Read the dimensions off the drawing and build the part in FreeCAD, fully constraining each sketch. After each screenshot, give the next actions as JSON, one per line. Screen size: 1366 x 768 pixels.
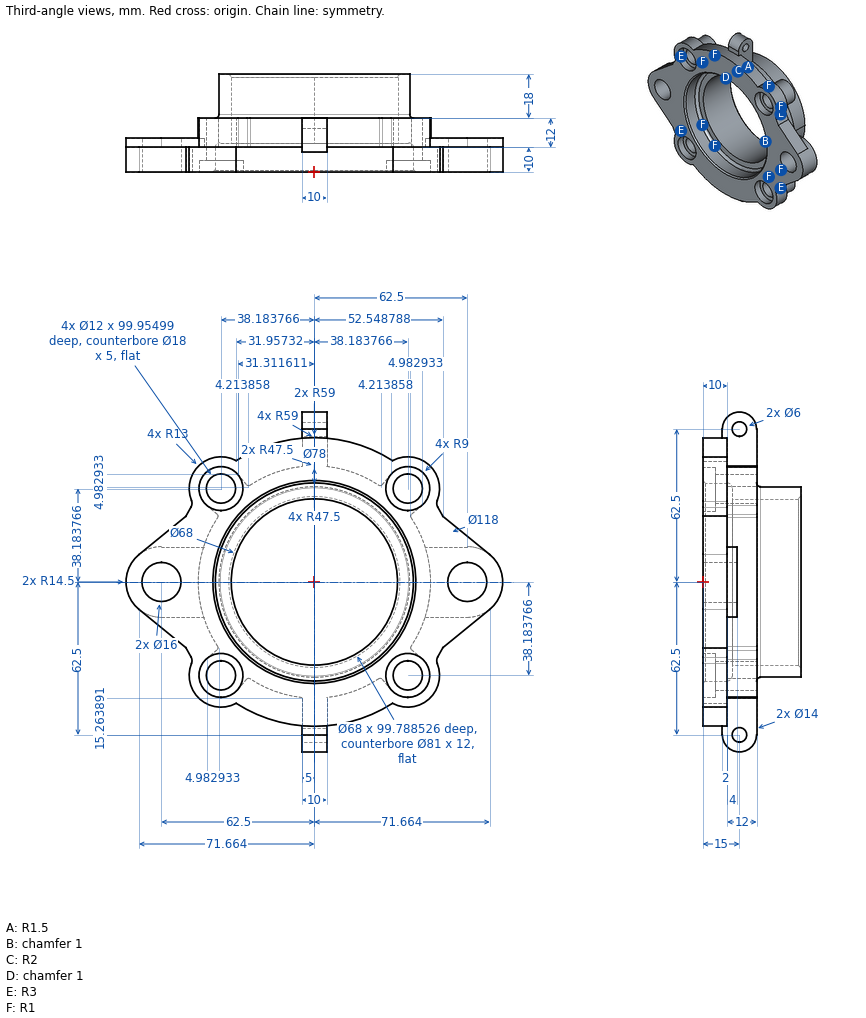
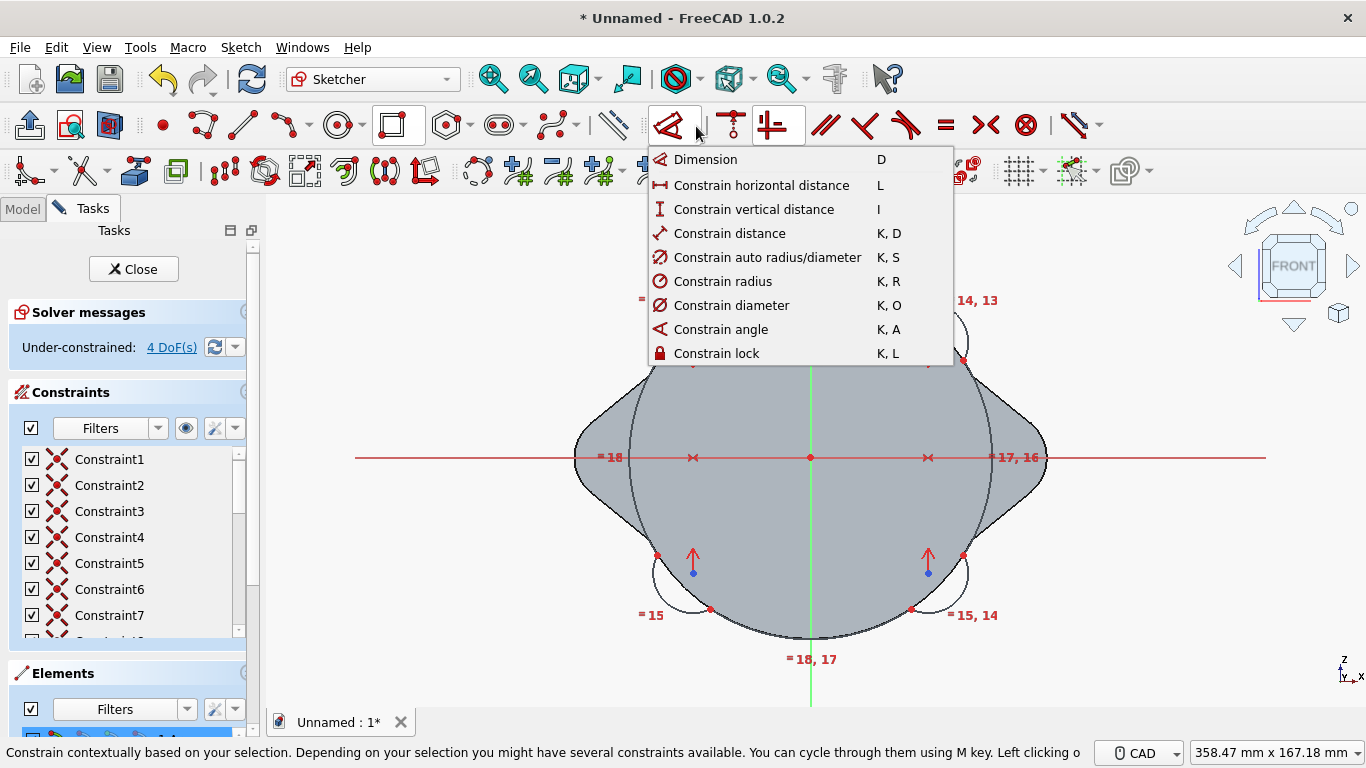
{"action": "left_click", "coordinate": [801, 281]}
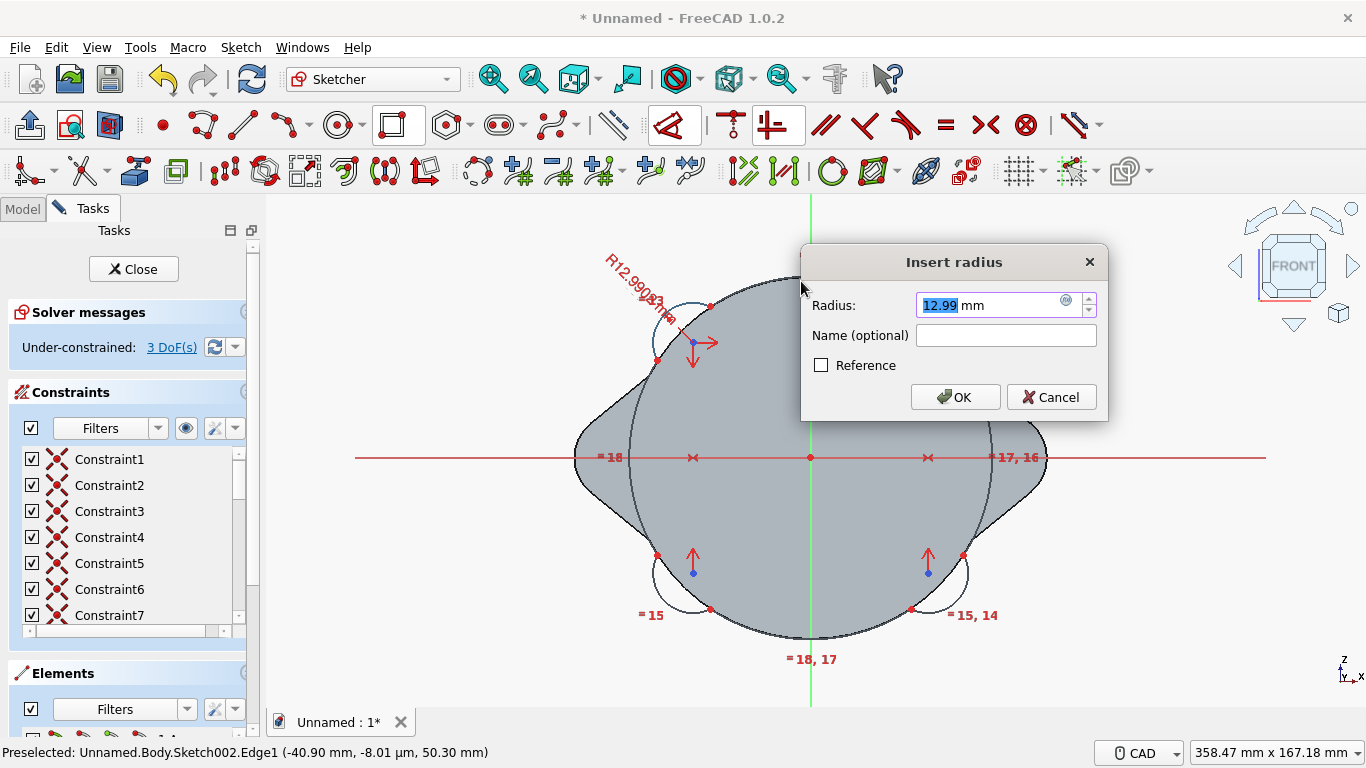
{"action": "type", "text": "13"}
{"action": "key", "text": "Return"}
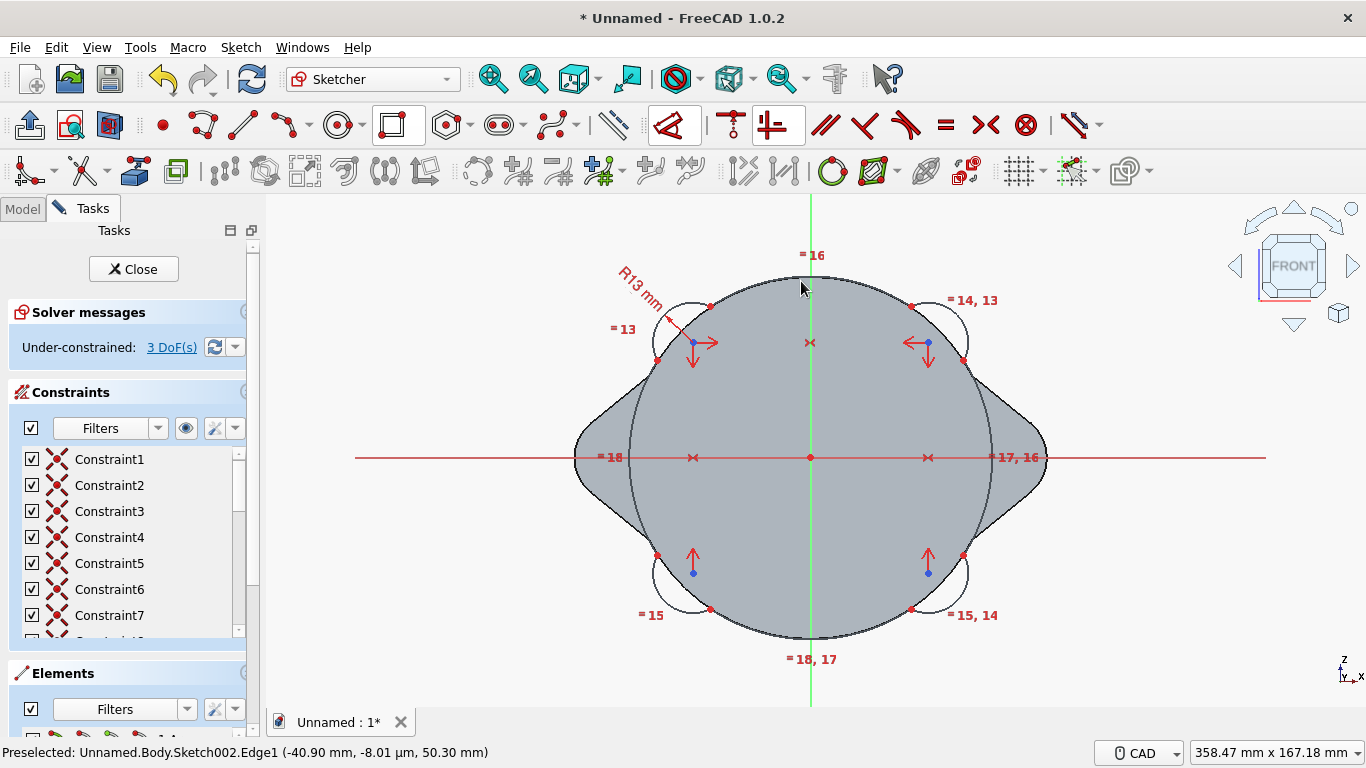
{"action": "left_click", "coordinate": [853, 281]}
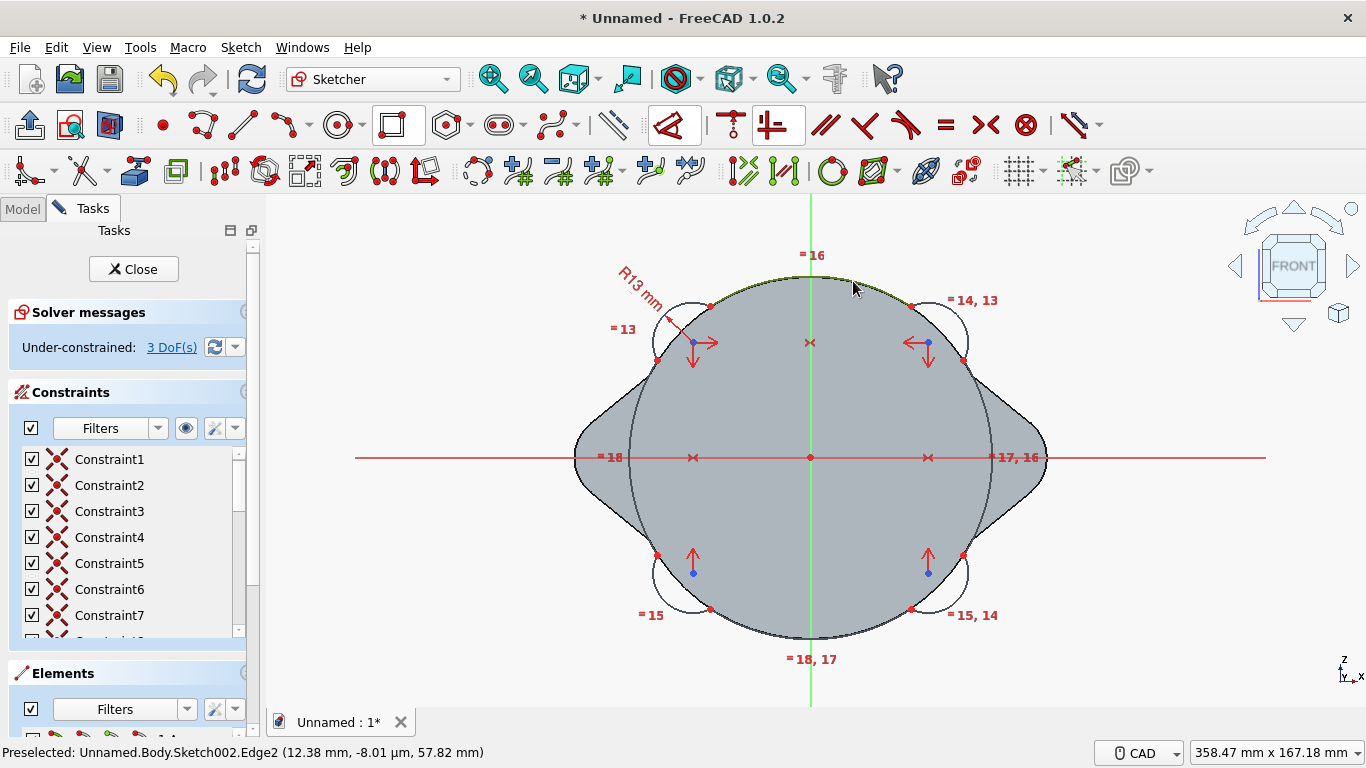
{"action": "left_click", "coordinate": [696, 126]}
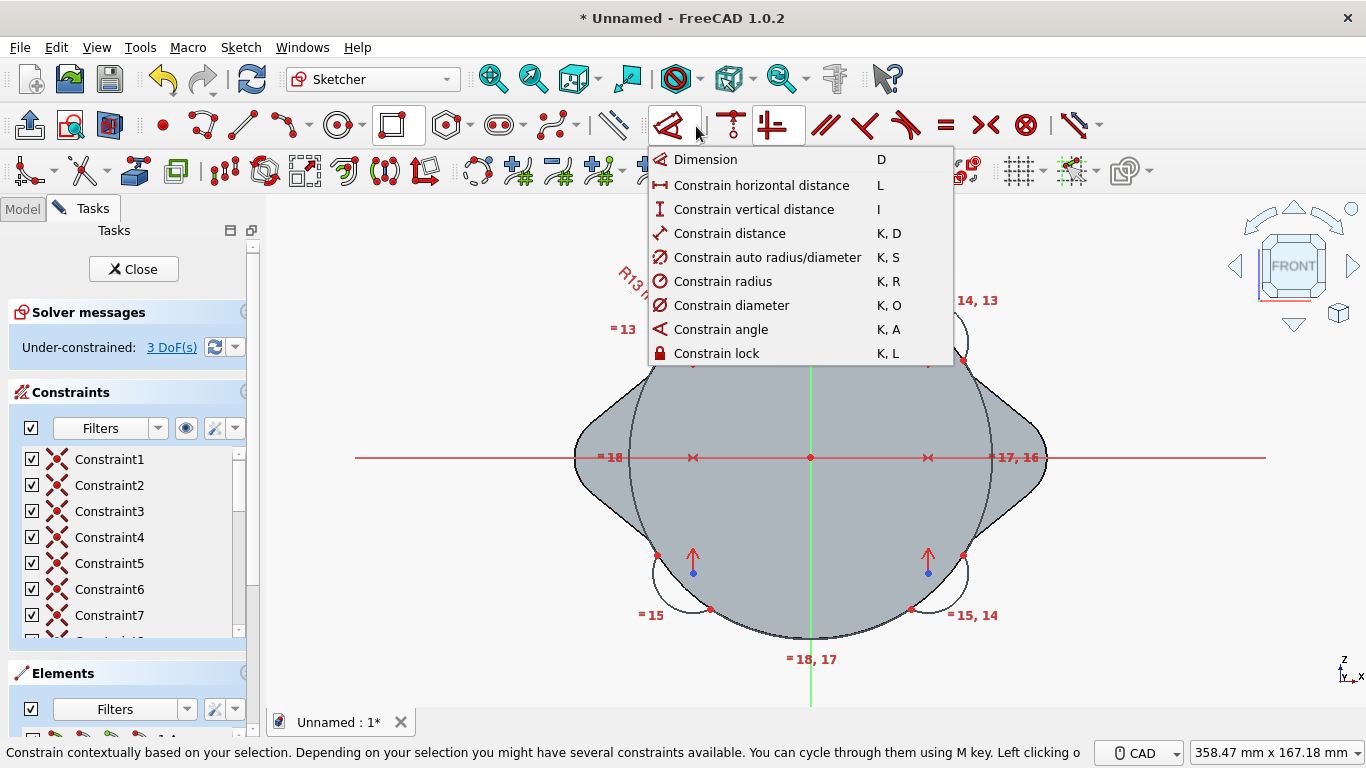
{"action": "left_click", "coordinate": [801, 281]}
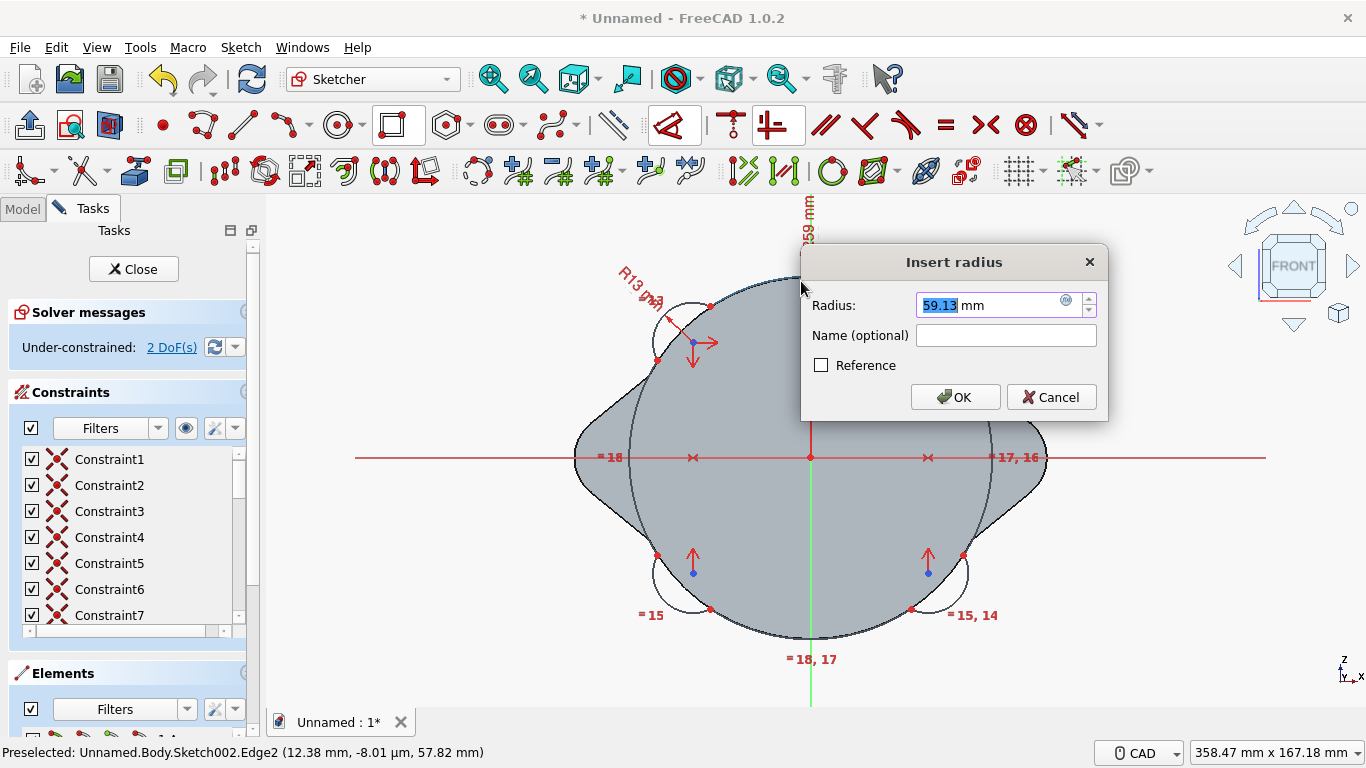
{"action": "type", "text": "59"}
{"action": "key", "text": "Return"}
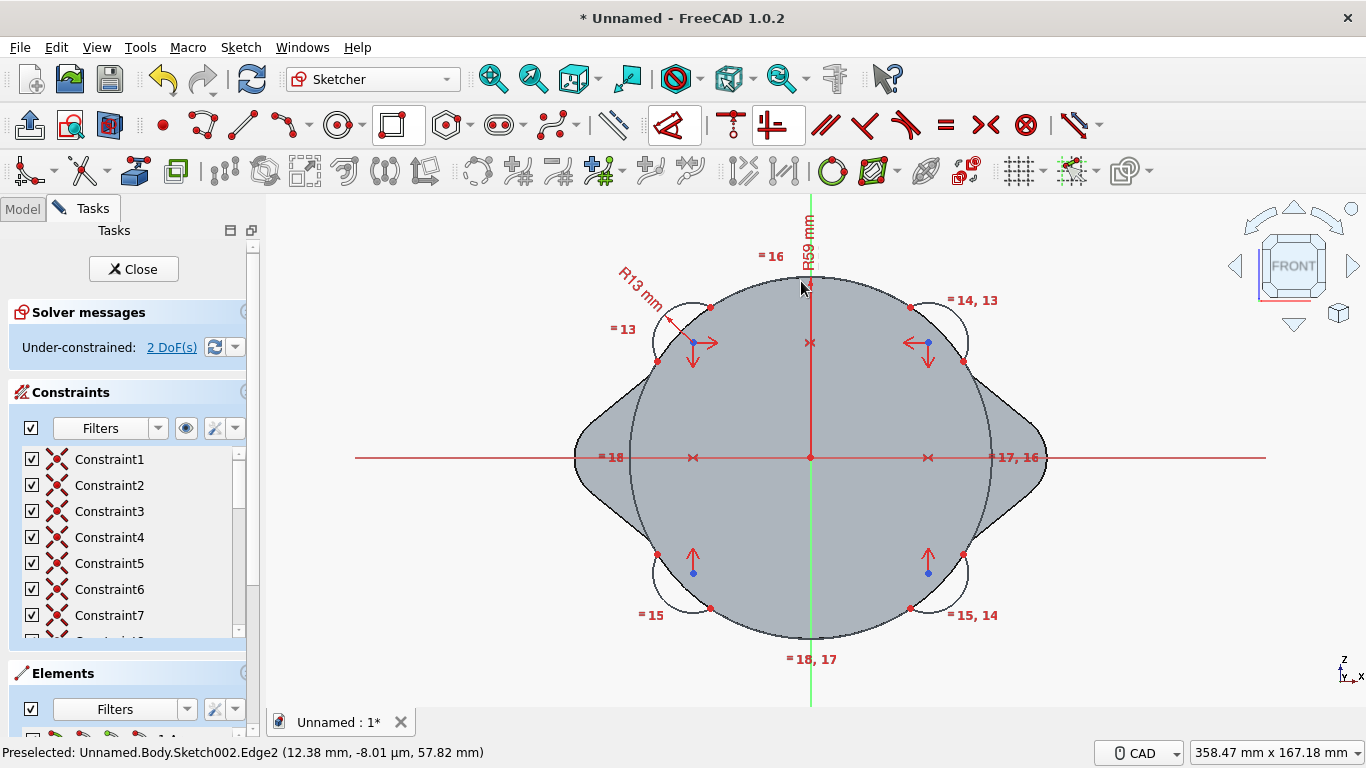
{"action": "left_click", "coordinate": [711, 307]}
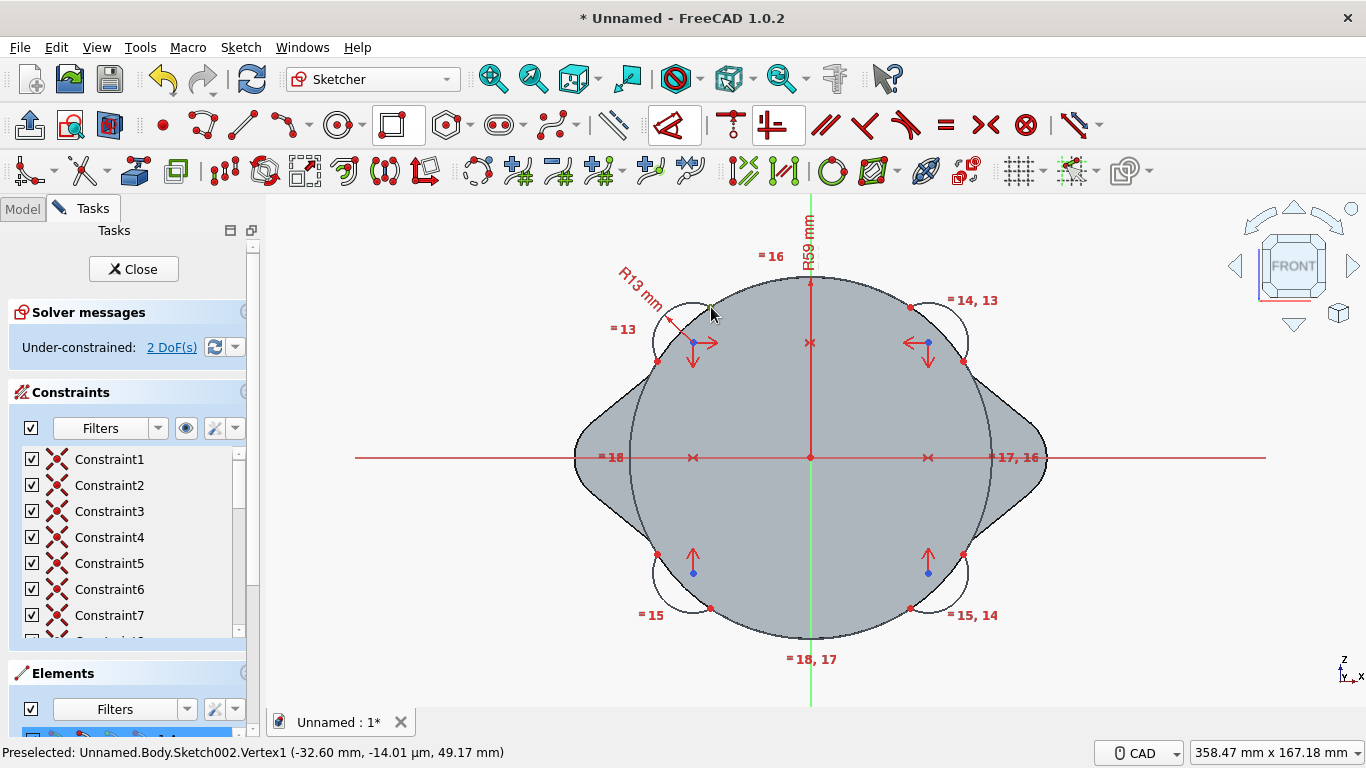
{"action": "key", "text": "l"}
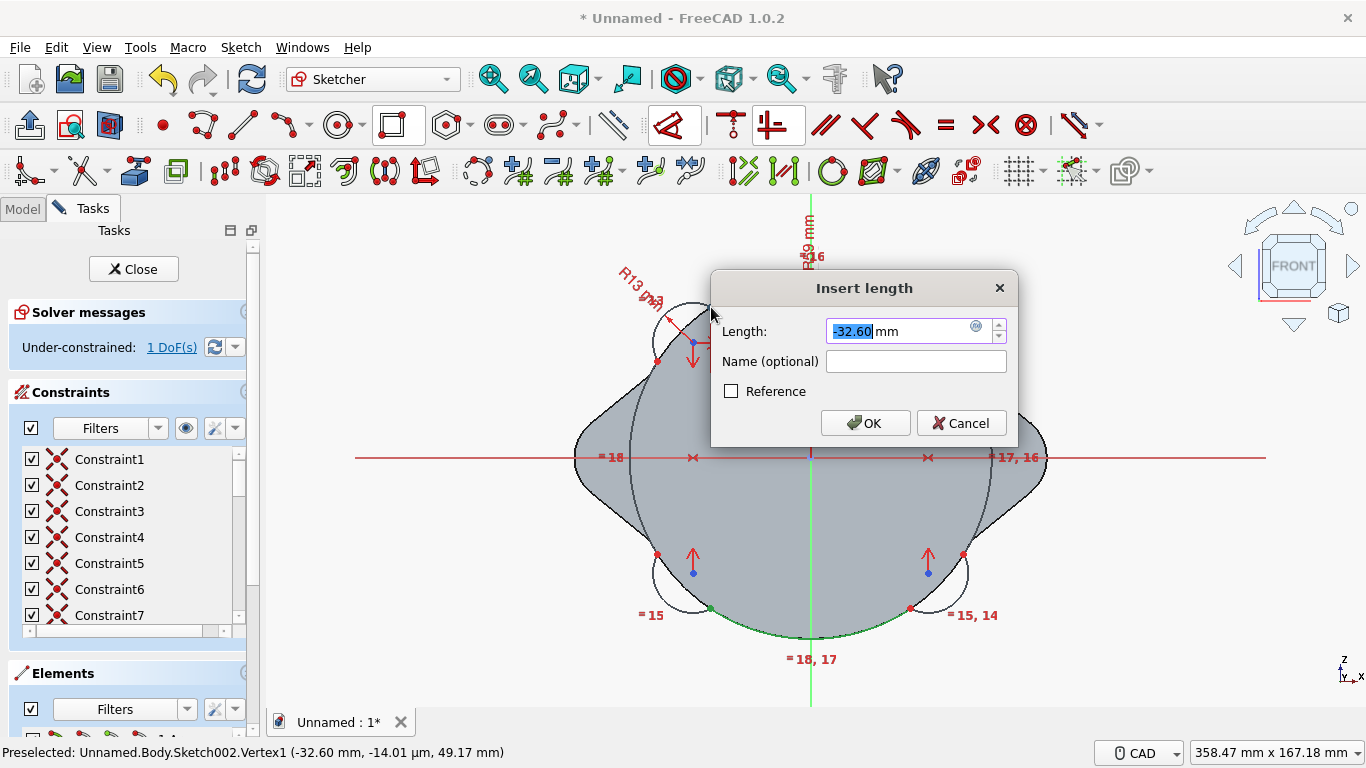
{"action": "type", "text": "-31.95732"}
{"action": "key", "text": "Return"}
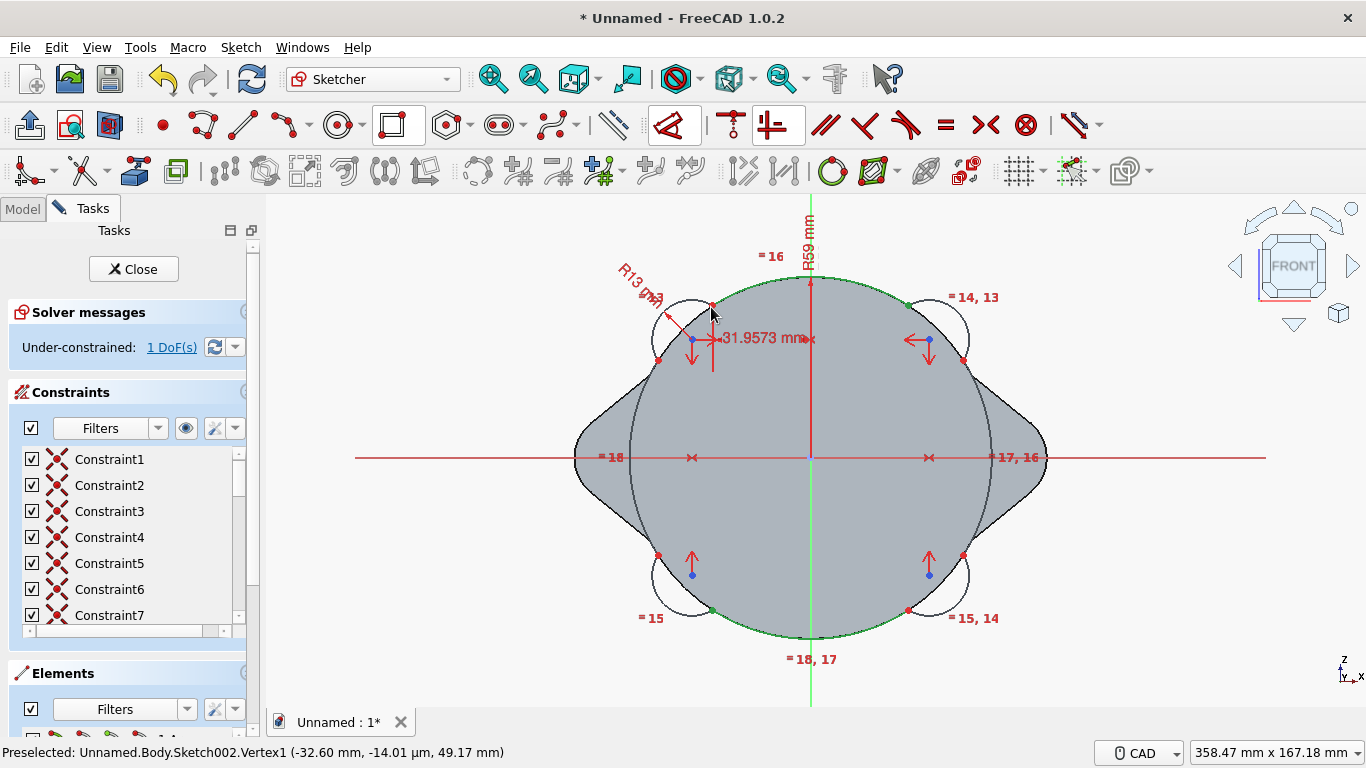
{"action": "left_click", "coordinate": [692, 340]}